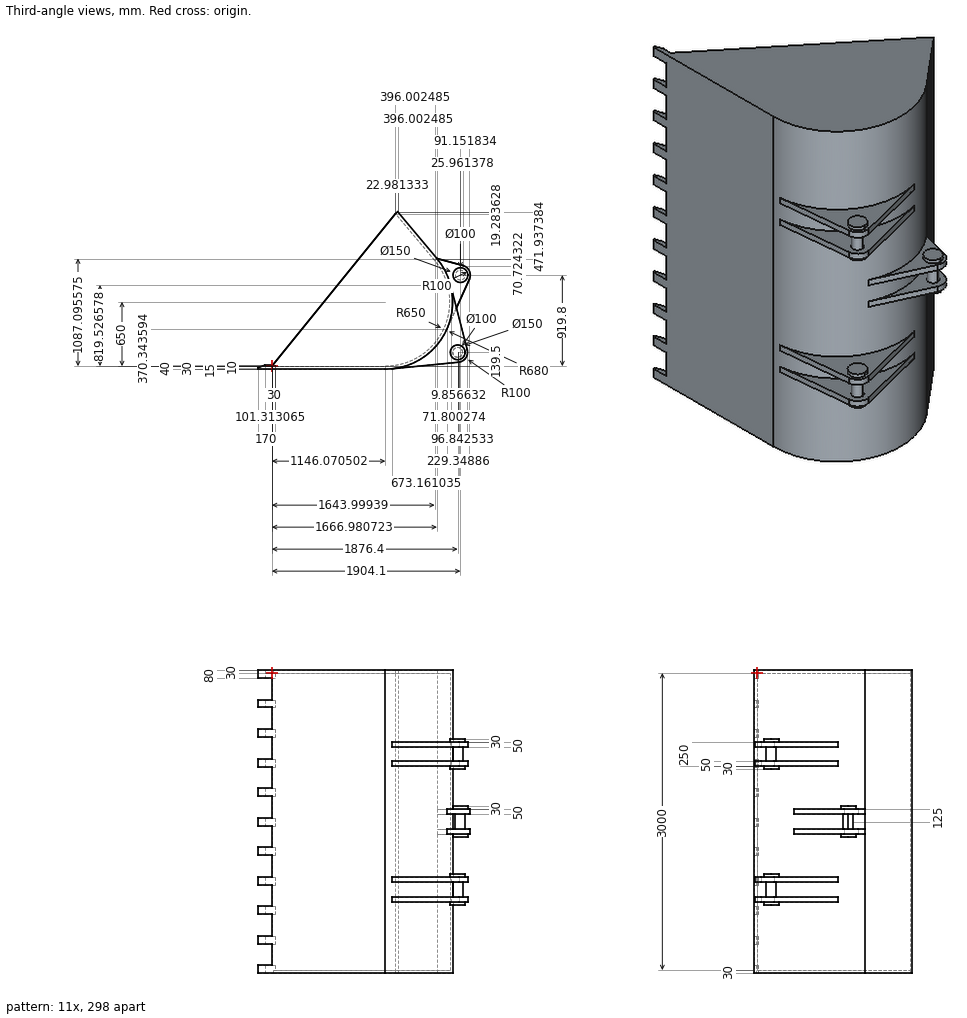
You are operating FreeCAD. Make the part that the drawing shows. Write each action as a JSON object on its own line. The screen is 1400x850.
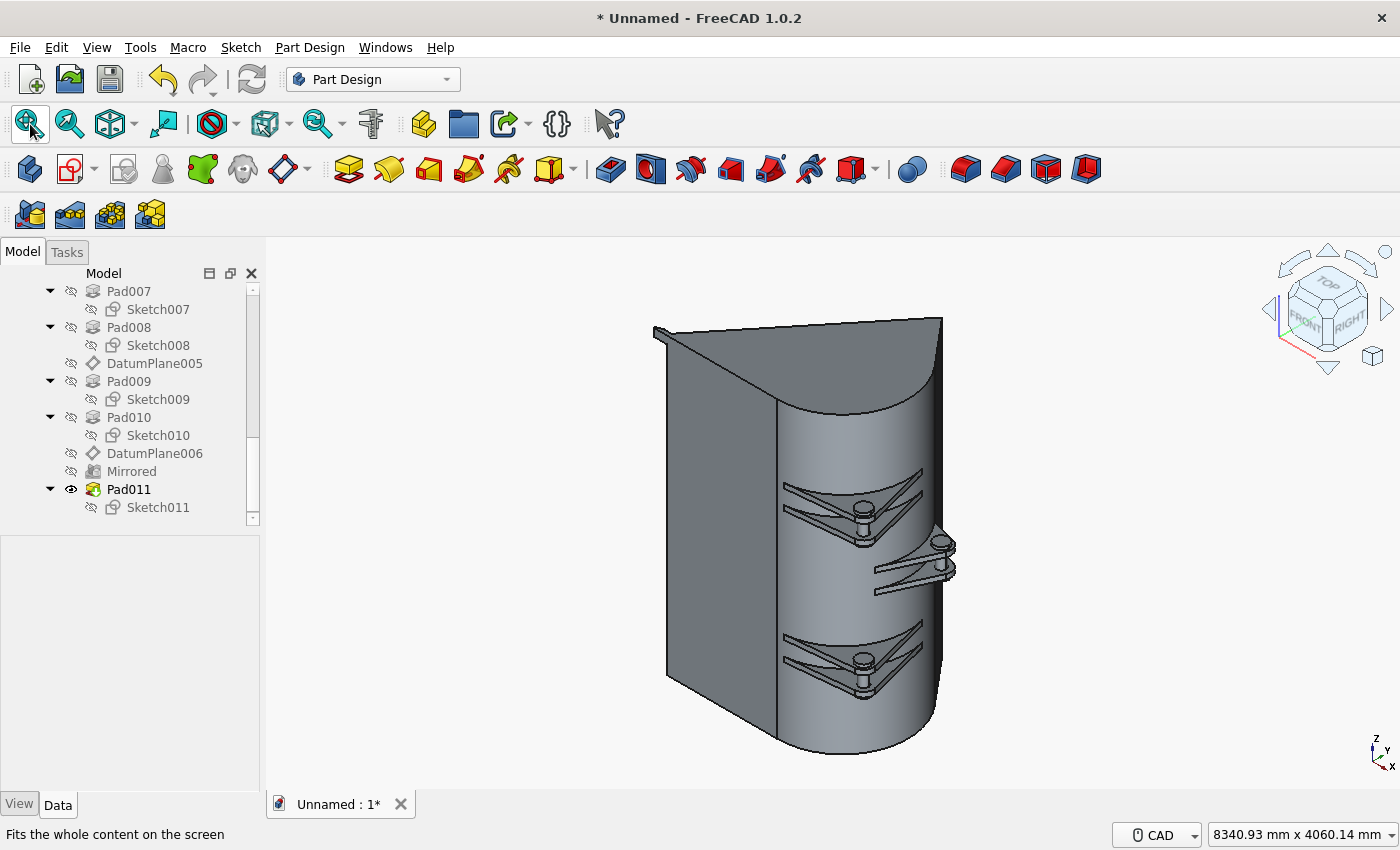
{"action": "left_click", "coordinate": [116, 489]}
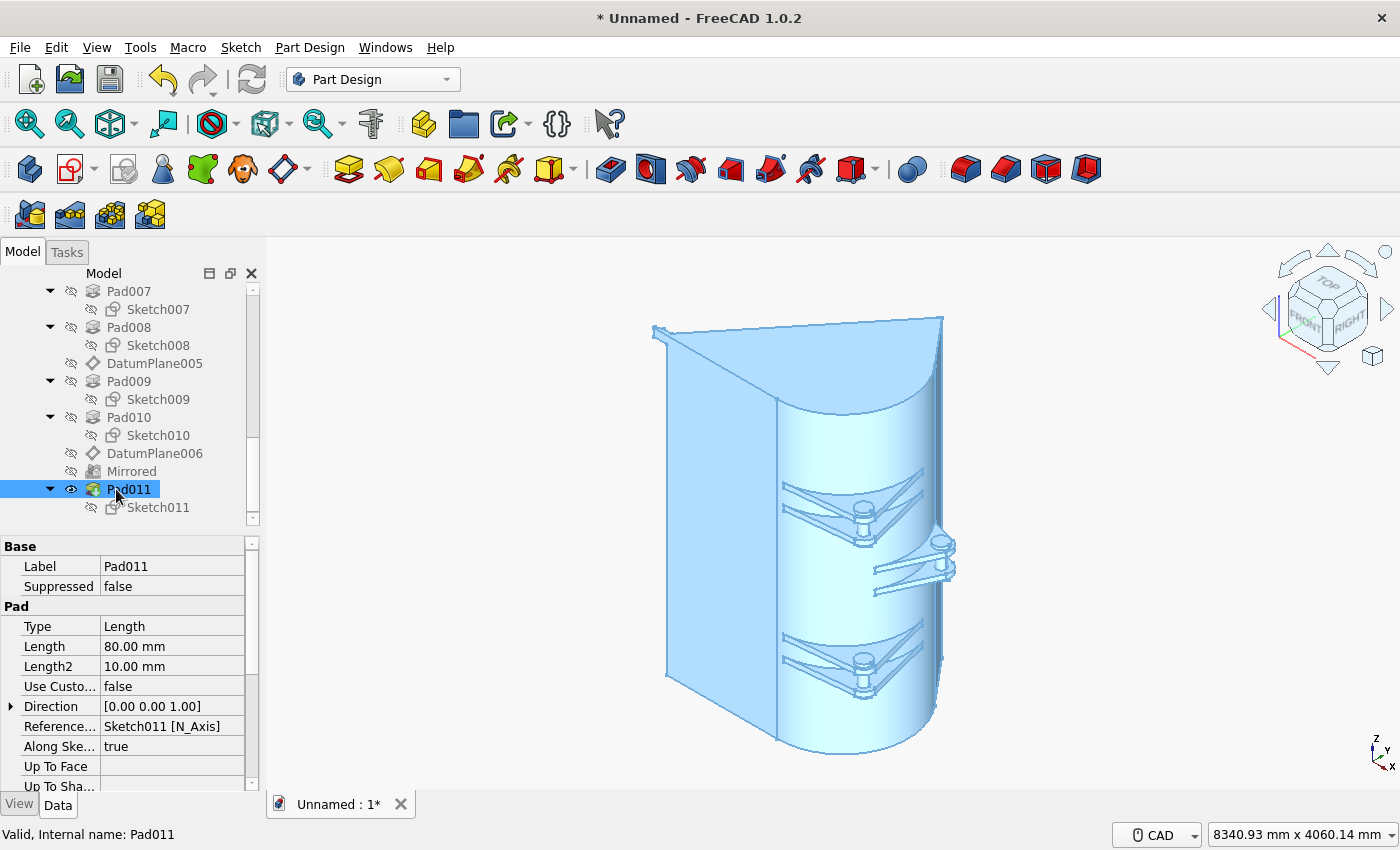
{"action": "left_click", "coordinate": [70, 214]}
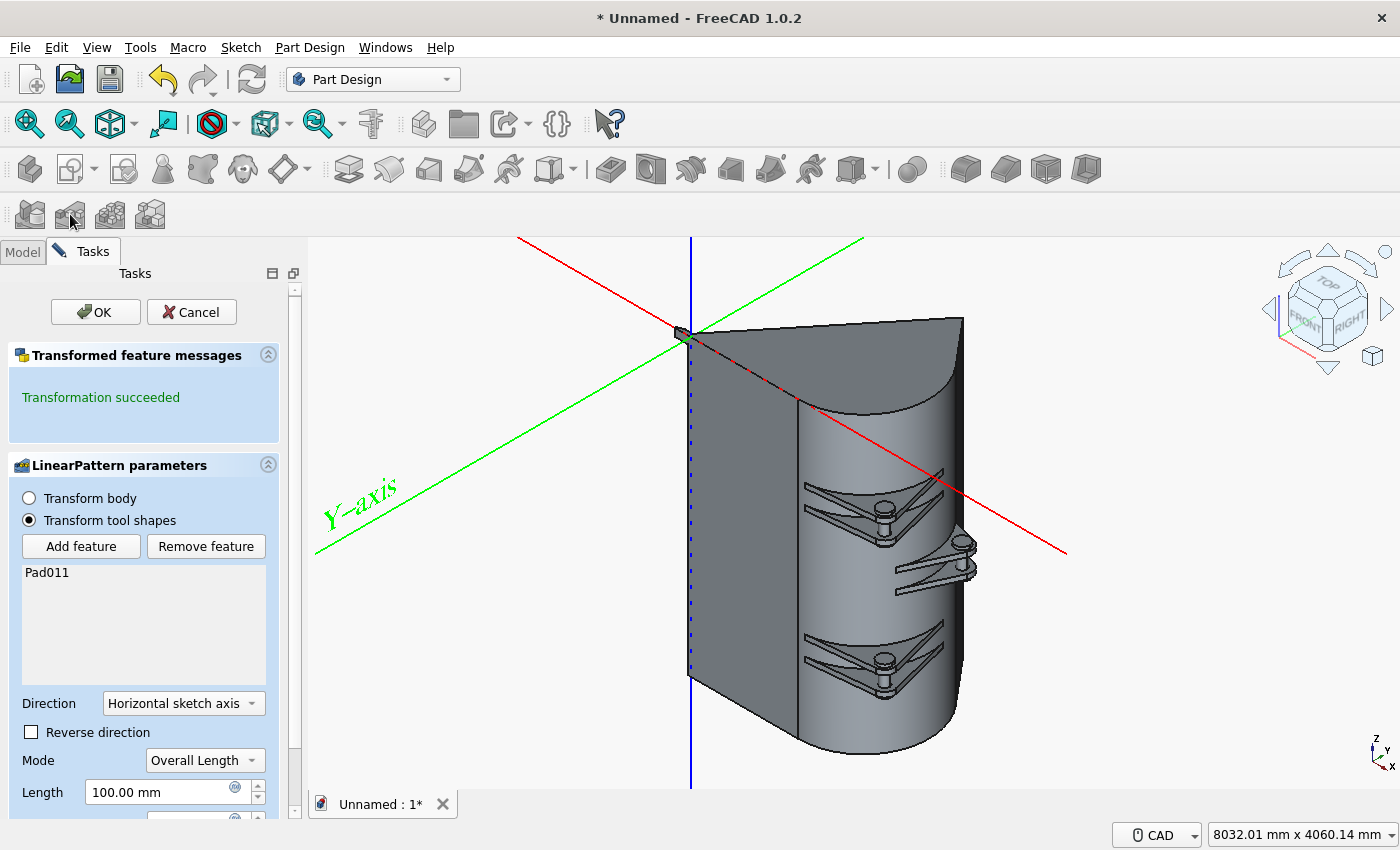
{"action": "left_click", "coordinate": [184, 704]}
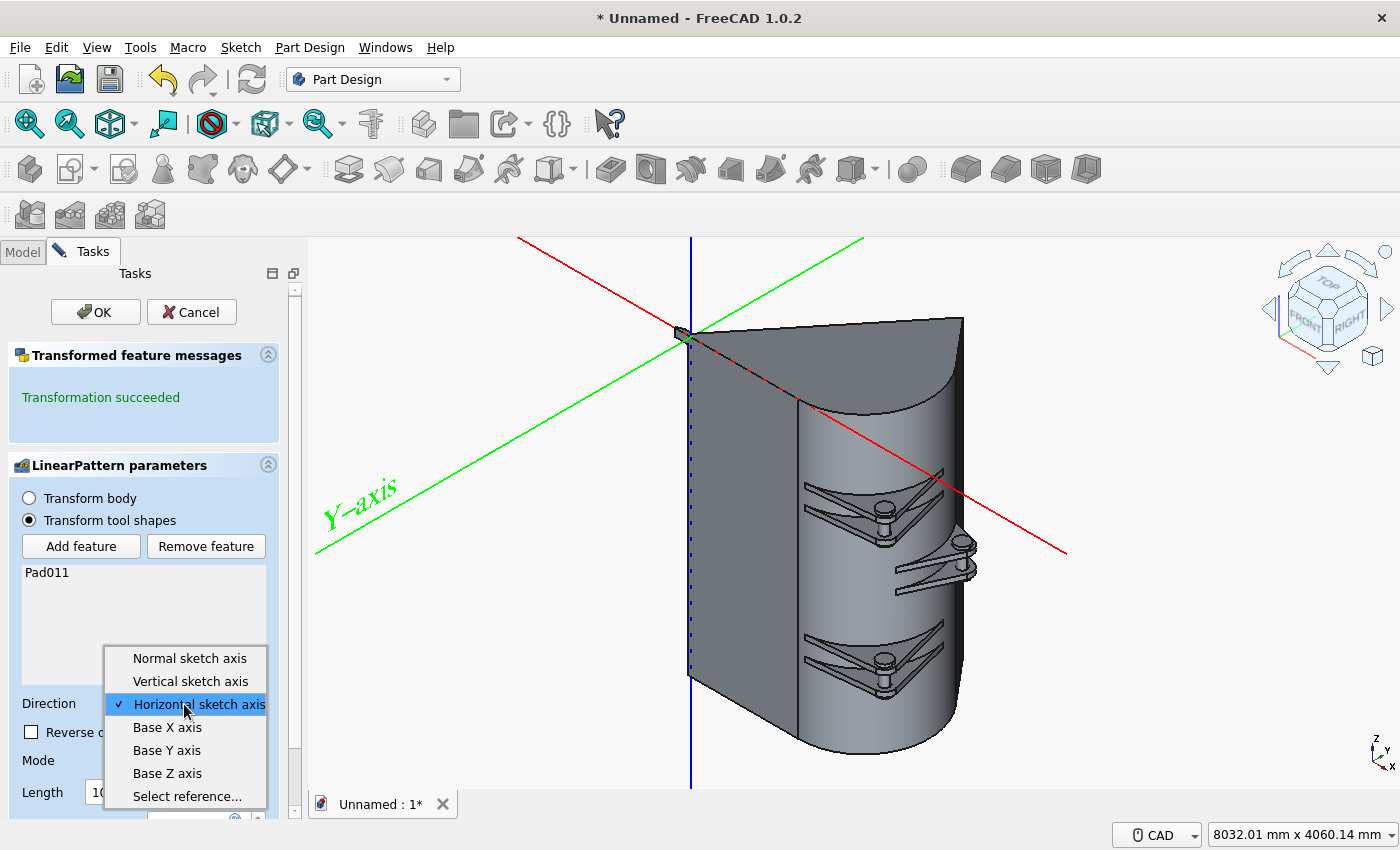
{"action": "left_click", "coordinate": [184, 774]}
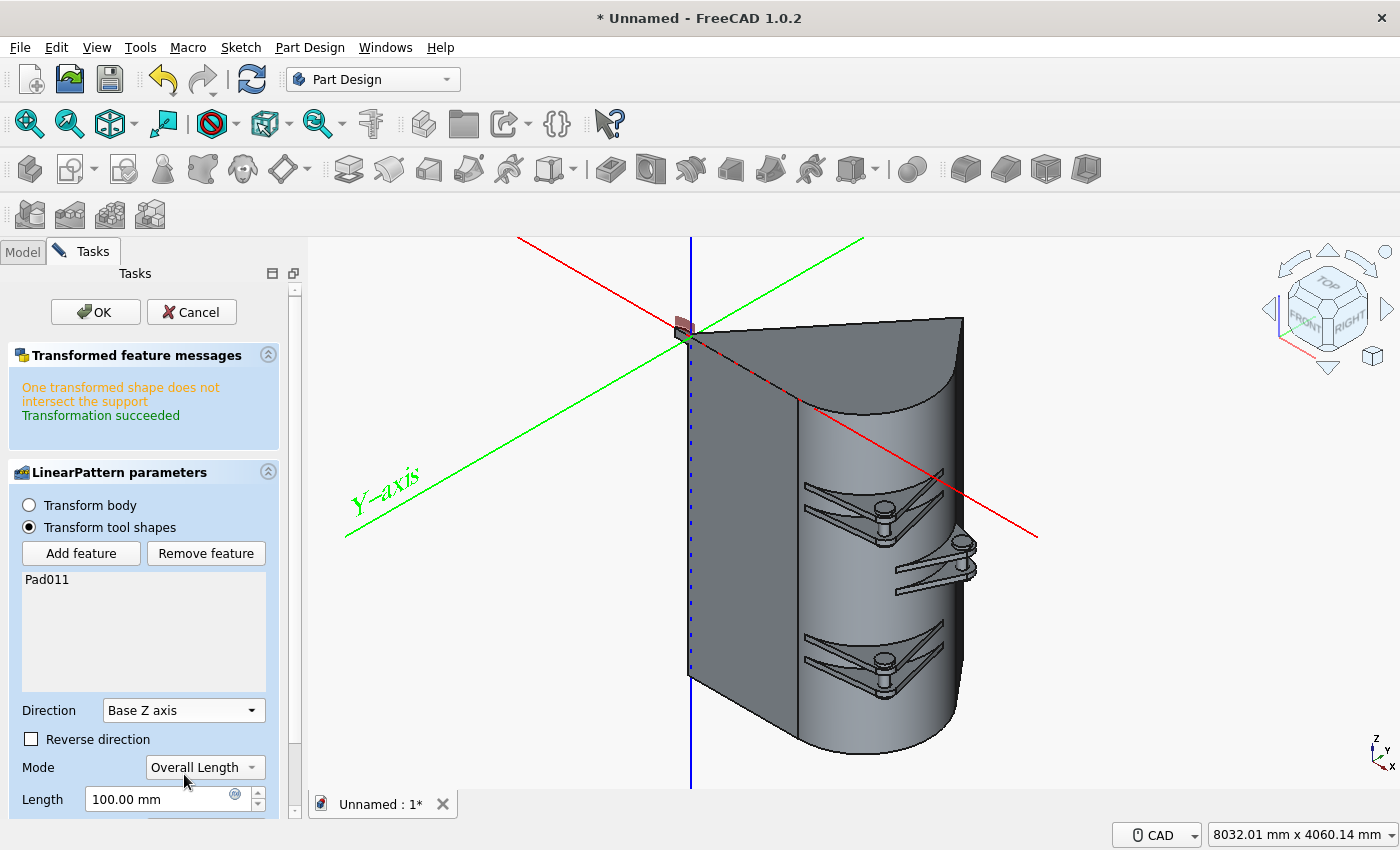
{"action": "left_click", "coordinate": [206, 768]}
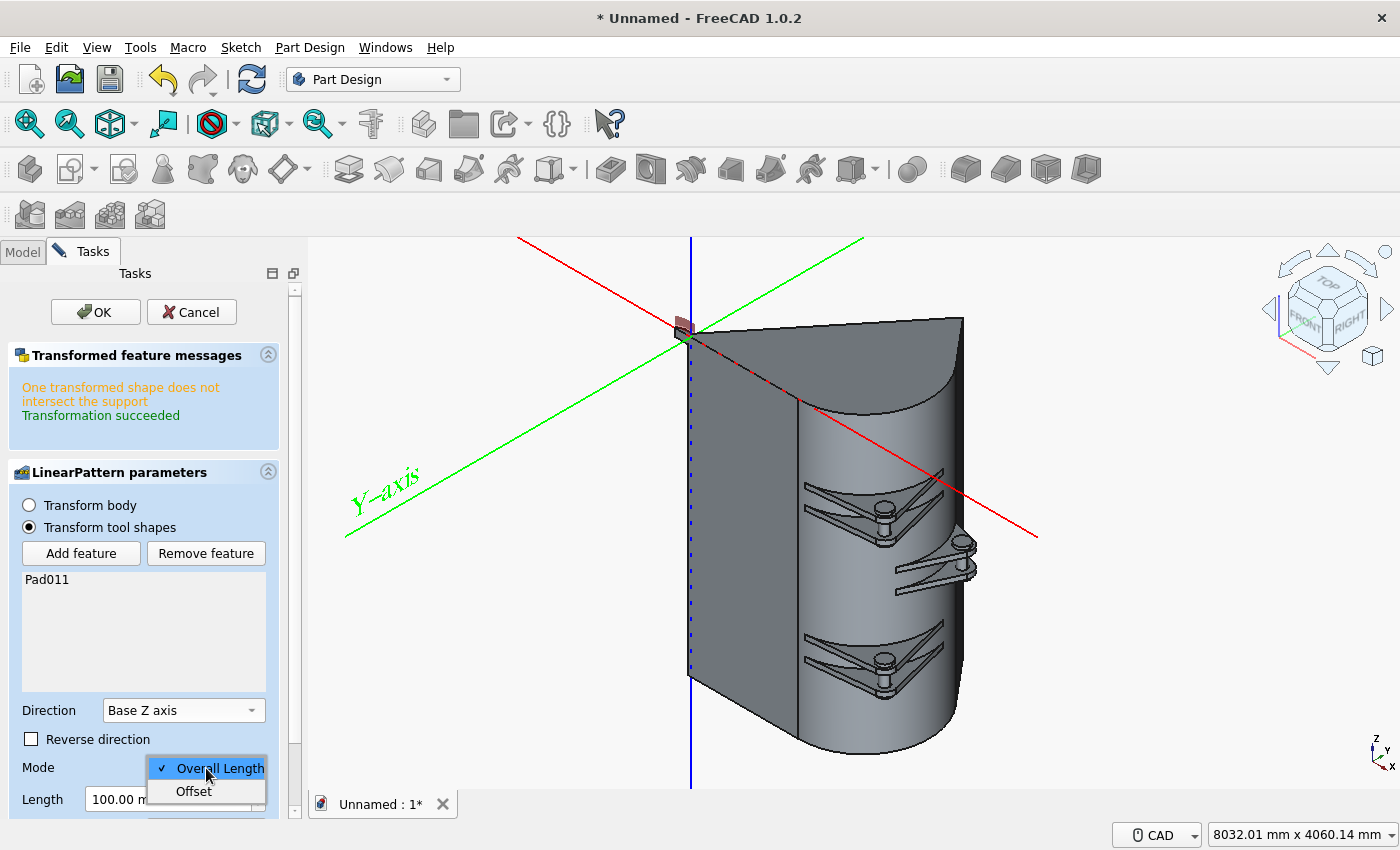
{"action": "left_click", "coordinate": [206, 792]}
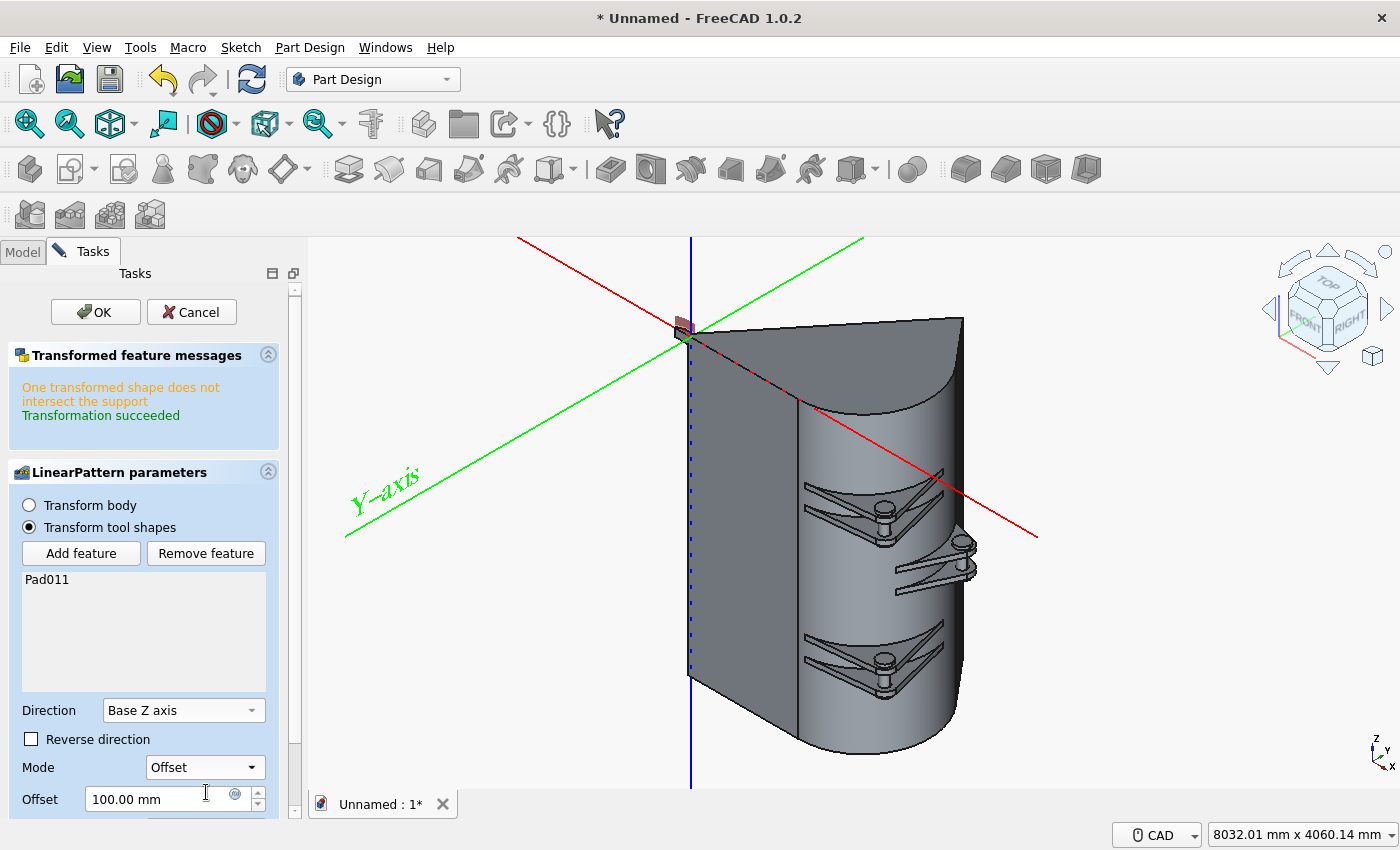
{"action": "triple_click", "coordinate": [168, 799]}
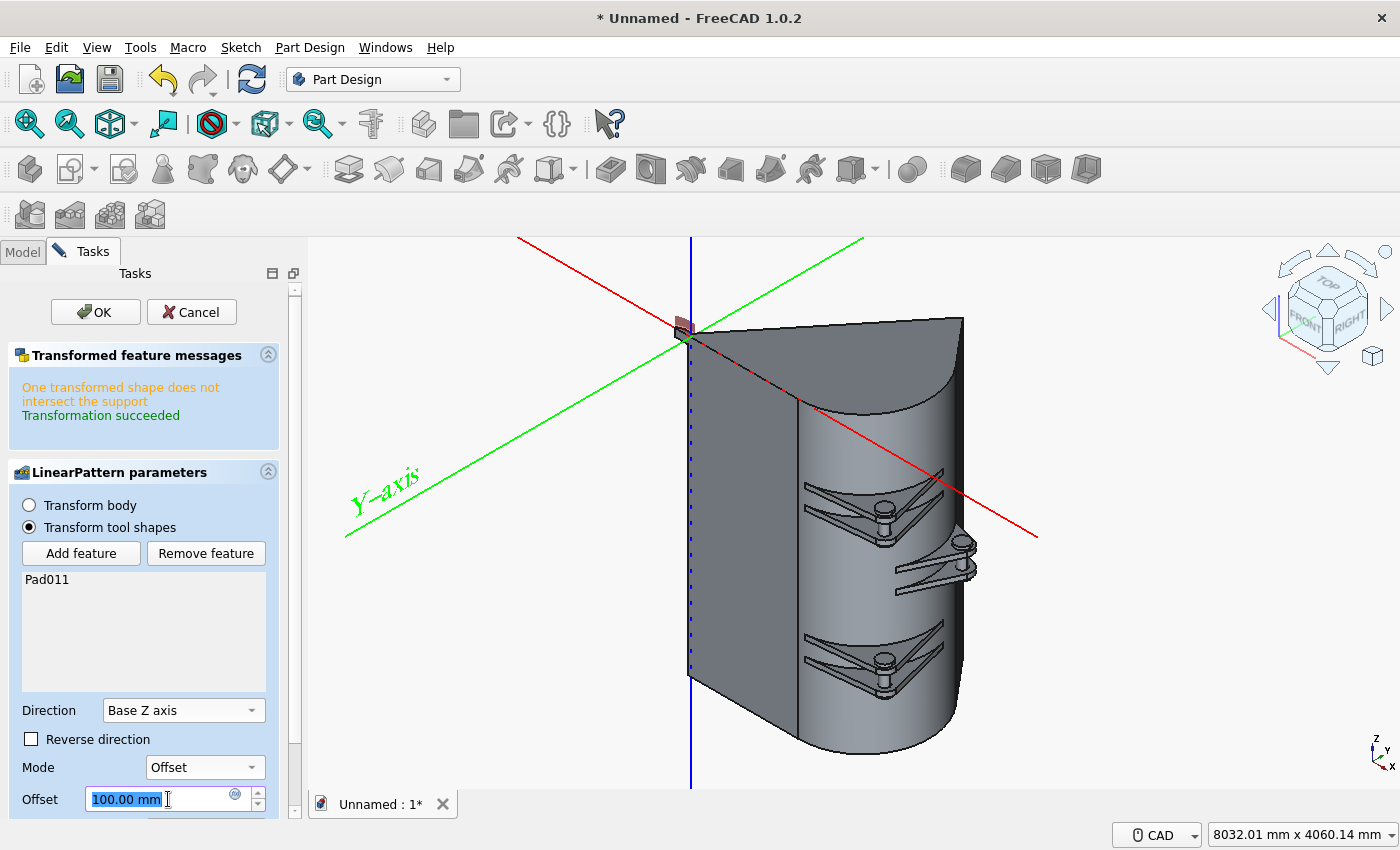
{"action": "type", "text": "298"}
{"action": "key", "text": "Tab"}